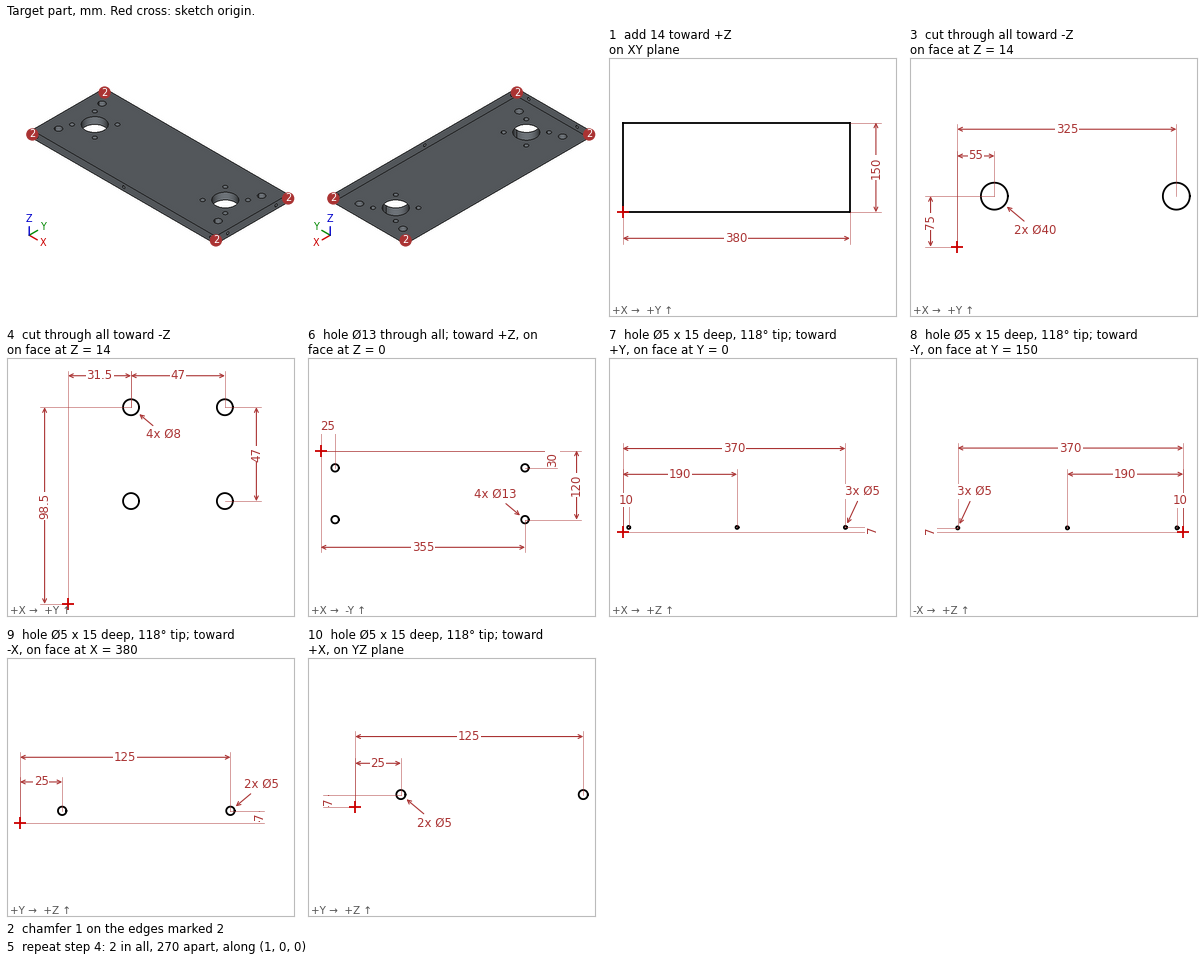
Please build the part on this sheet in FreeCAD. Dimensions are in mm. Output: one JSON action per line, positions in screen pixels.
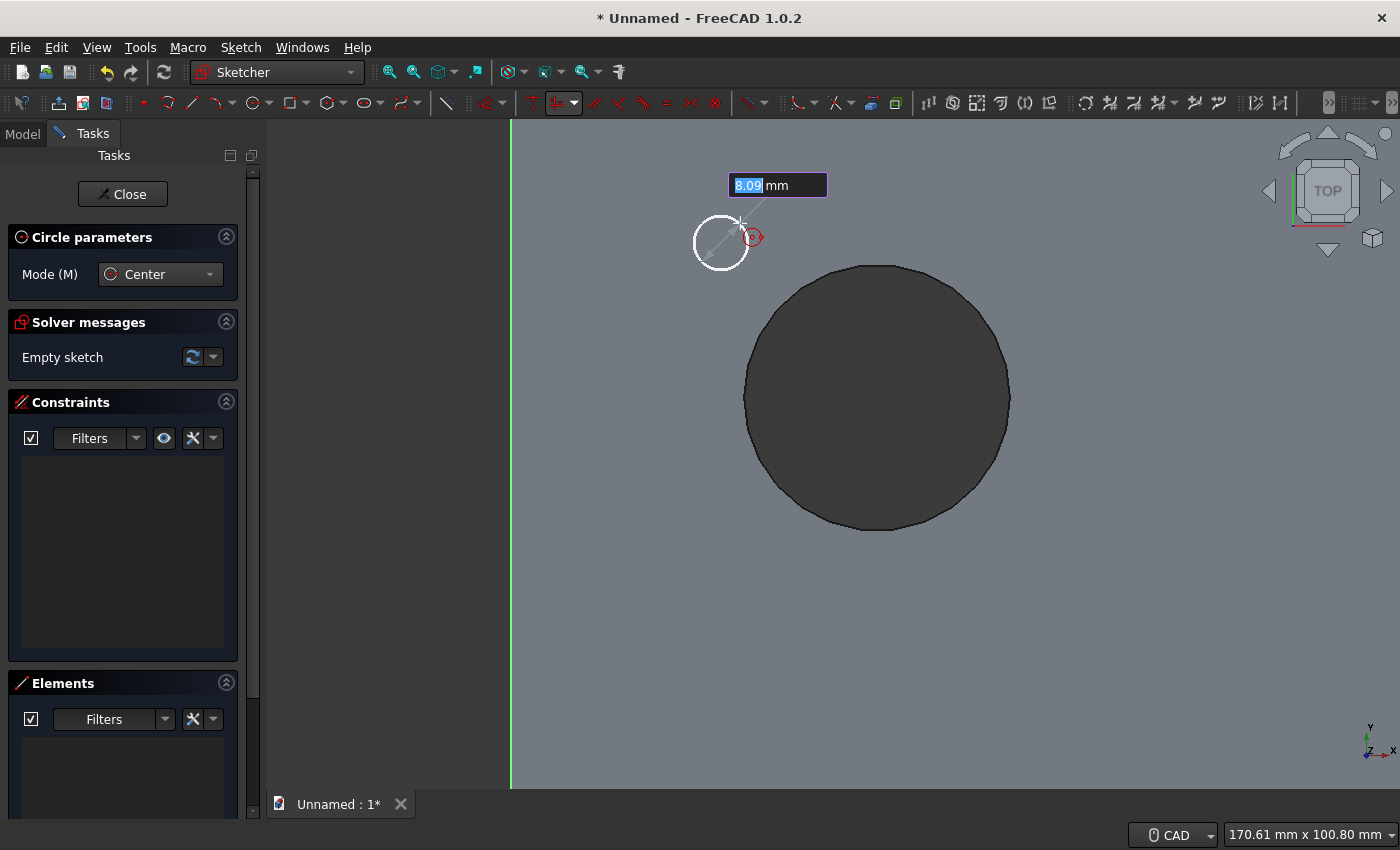
{"action": "type", "text": "8"}
{"action": "key", "text": "Return"}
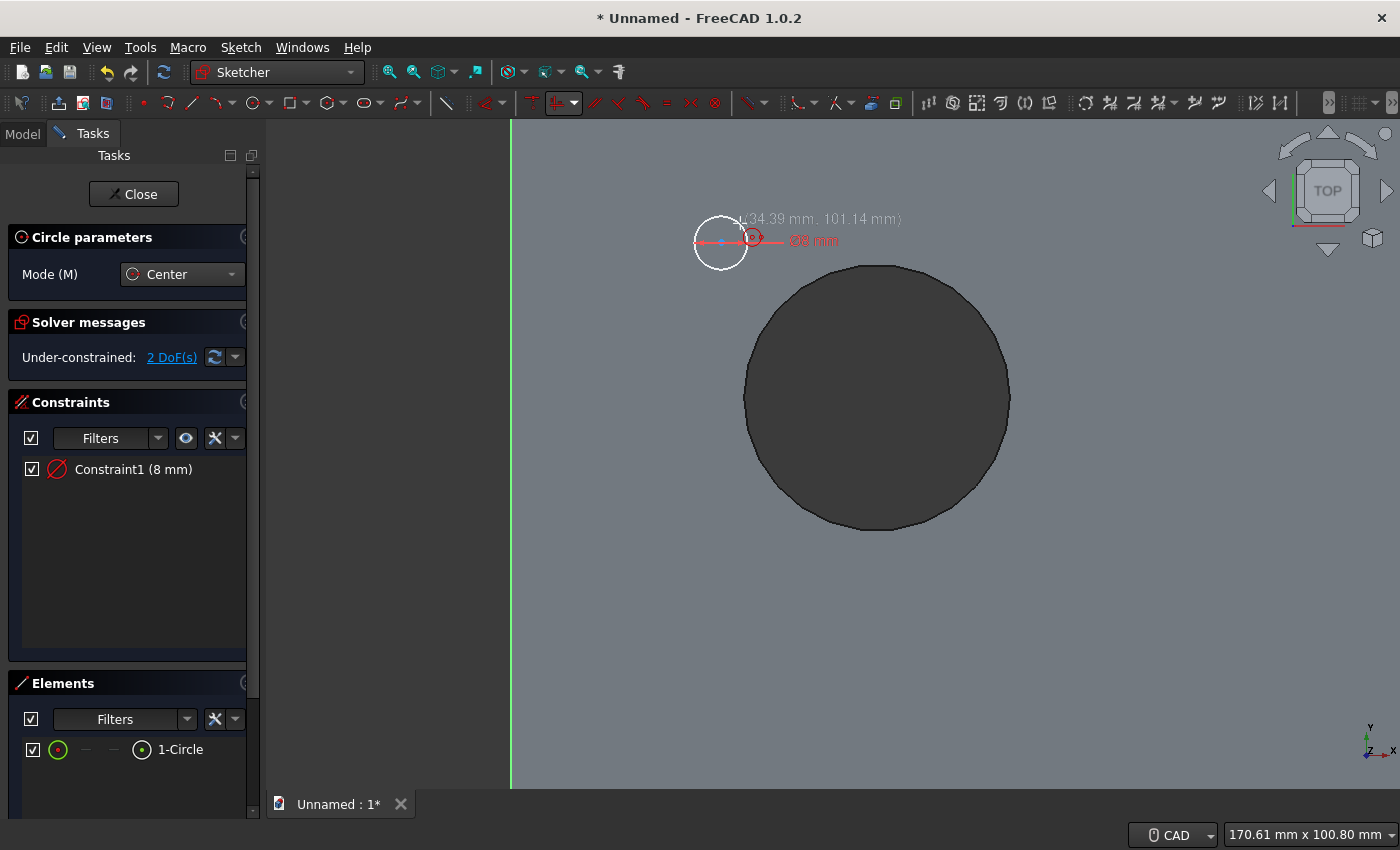
{"action": "left_click", "coordinate": [1033, 242]}
{"action": "mouse_move", "coordinate": [1052, 223]}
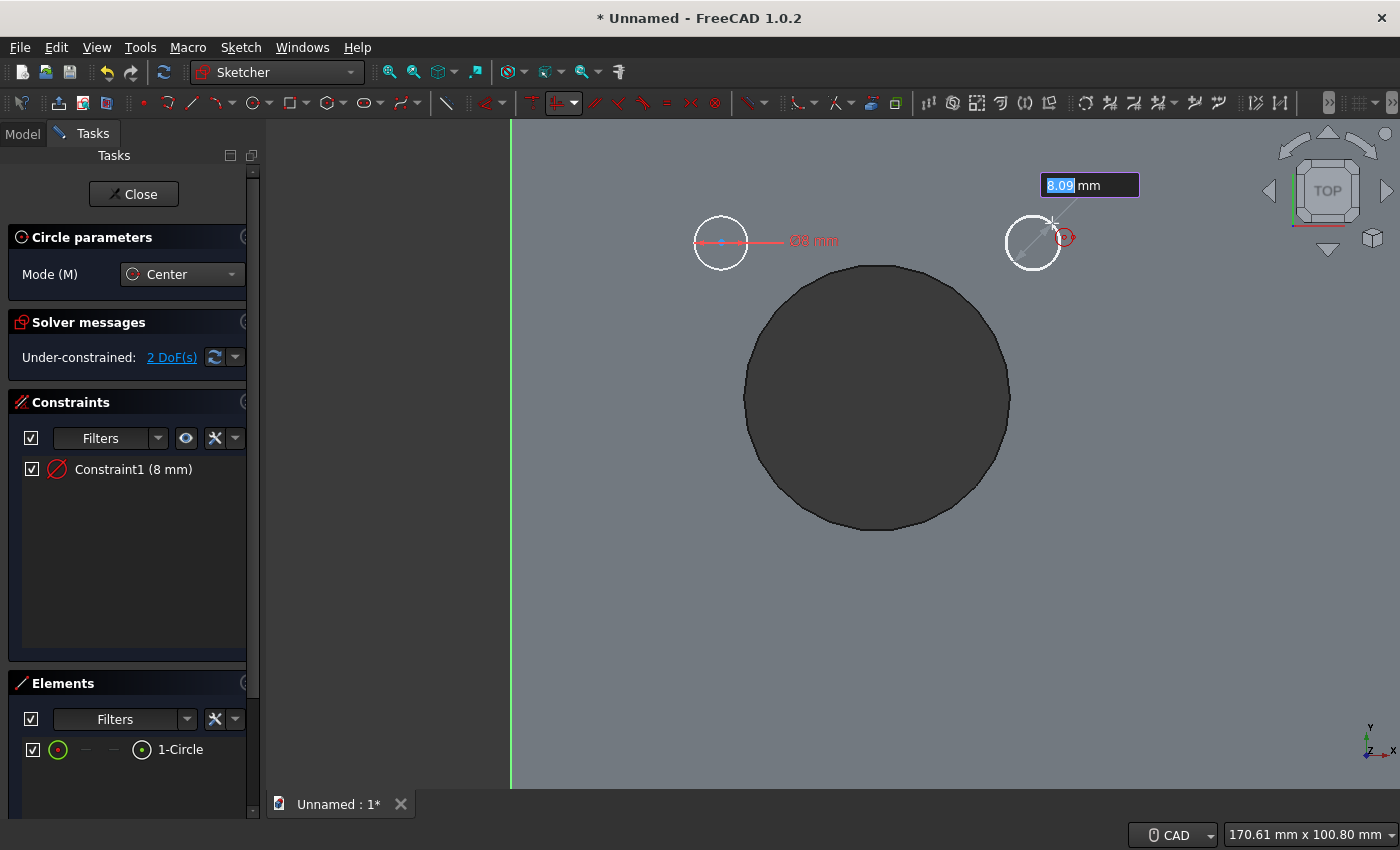
{"action": "type", "text": "8"}
{"action": "key", "text": "Return"}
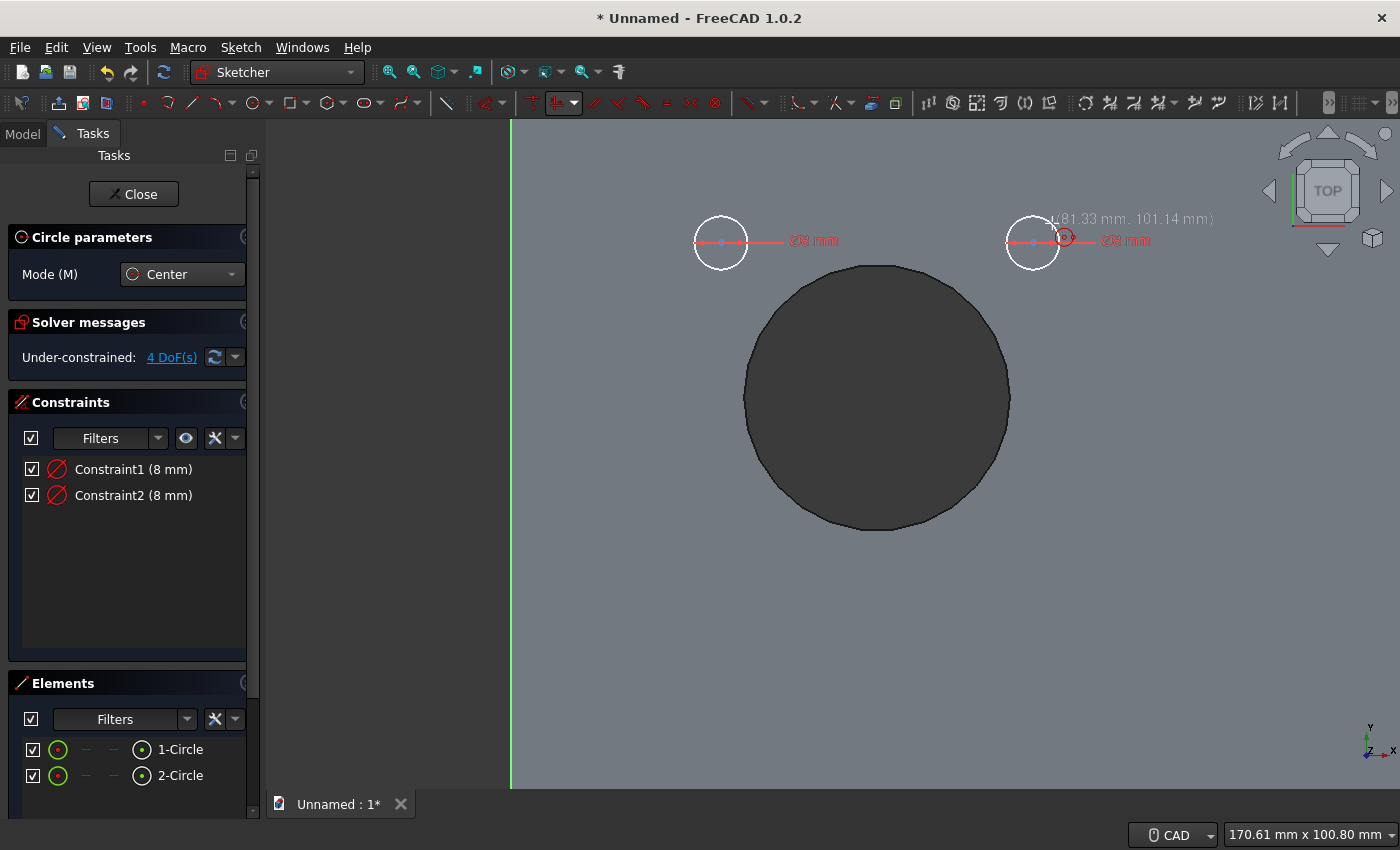
{"action": "left_click", "coordinate": [1033, 554]}
{"action": "mouse_move", "coordinate": [1052, 535]}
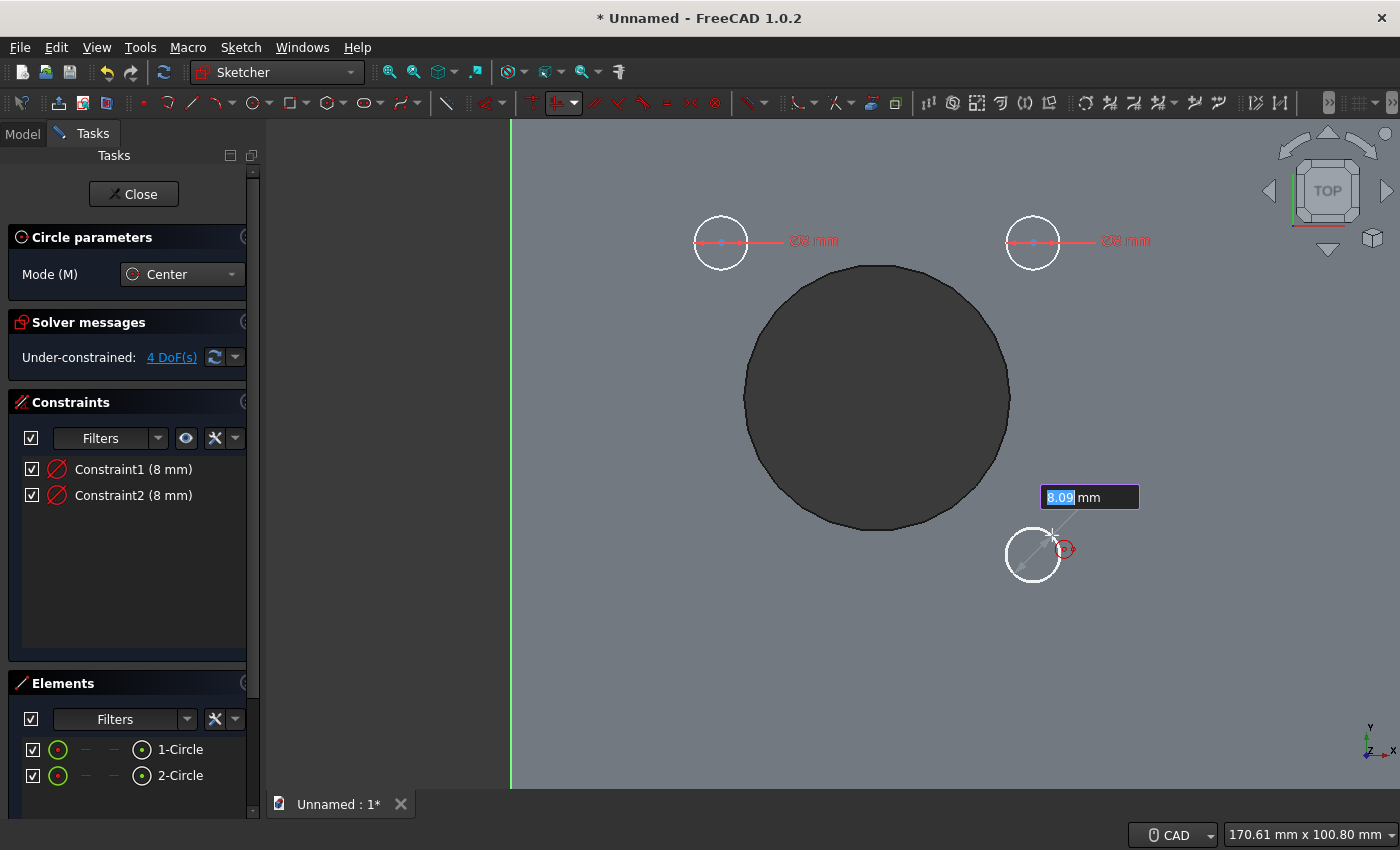
{"action": "type", "text": "8"}
{"action": "key", "text": "Return"}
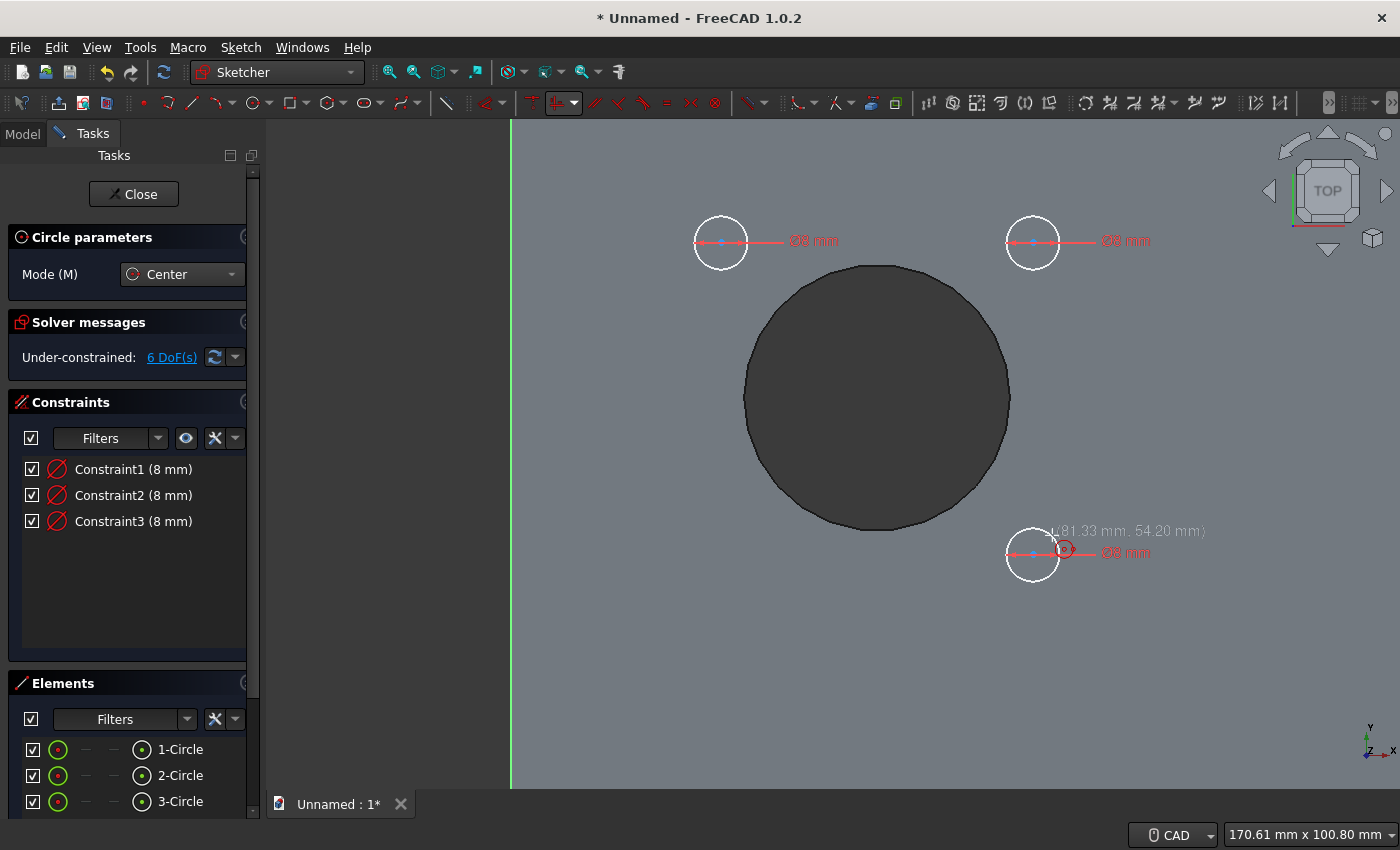
{"action": "left_click", "coordinate": [721, 554]}
{"action": "mouse_move", "coordinate": [740, 535]}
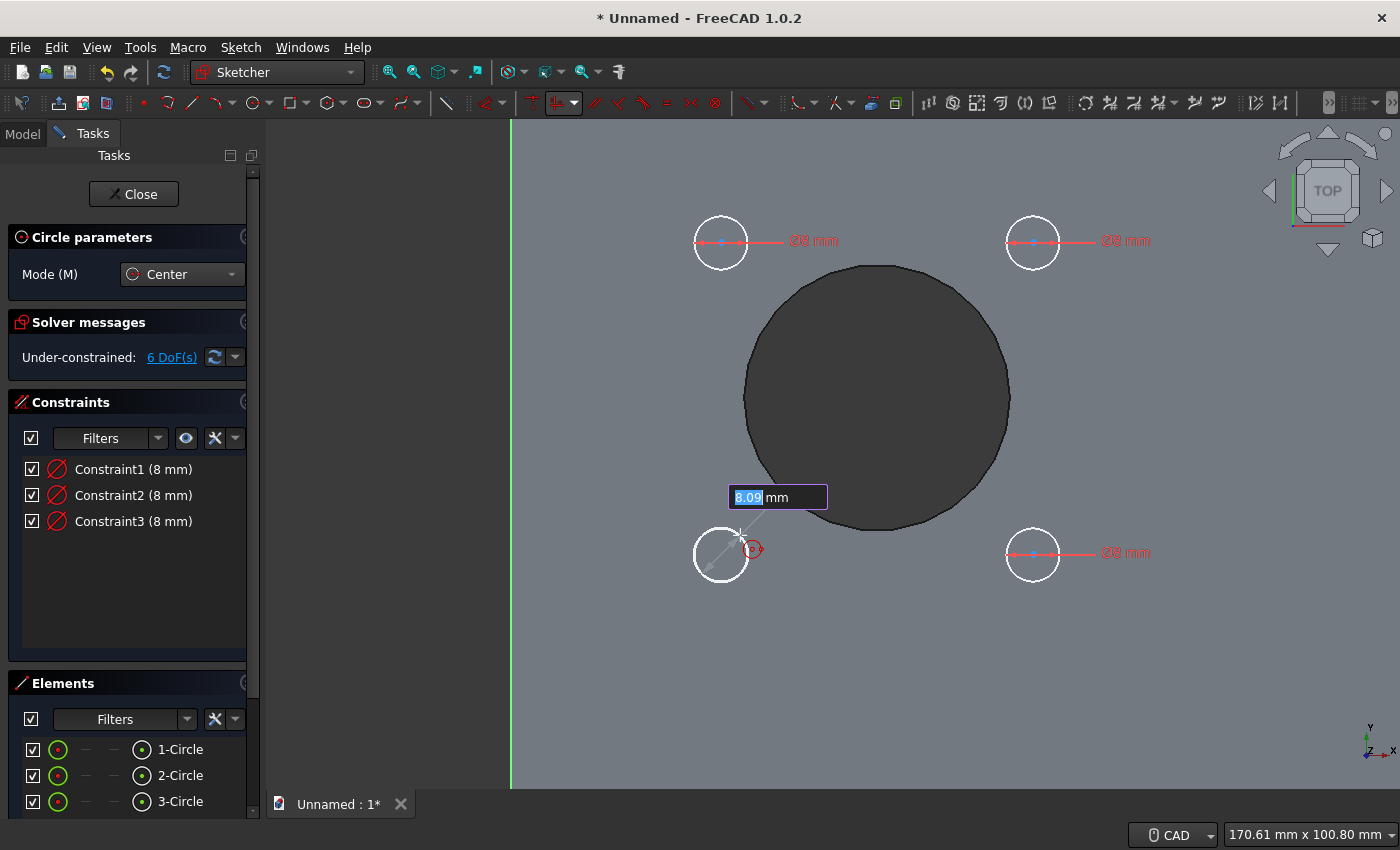
{"action": "type", "text": "8"}
{"action": "key", "text": "Return"}
{"action": "key", "text": "Escape"}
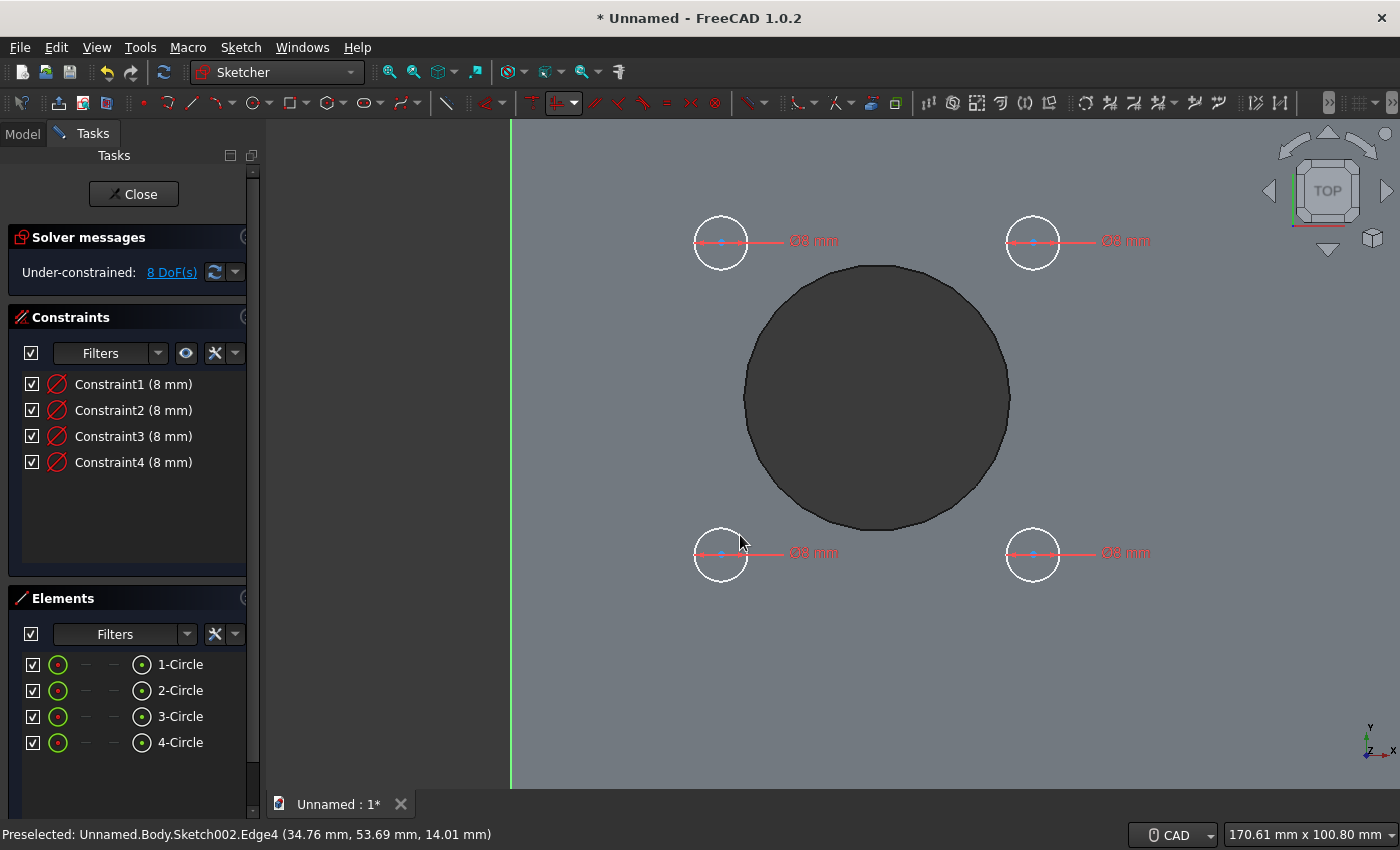
{"action": "left_click", "coordinate": [721, 243]}